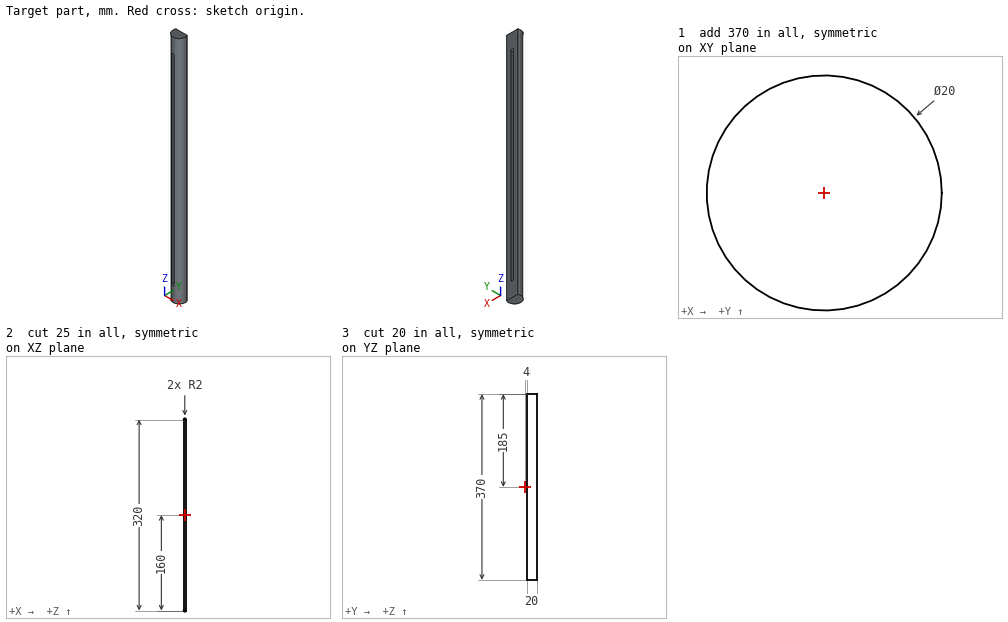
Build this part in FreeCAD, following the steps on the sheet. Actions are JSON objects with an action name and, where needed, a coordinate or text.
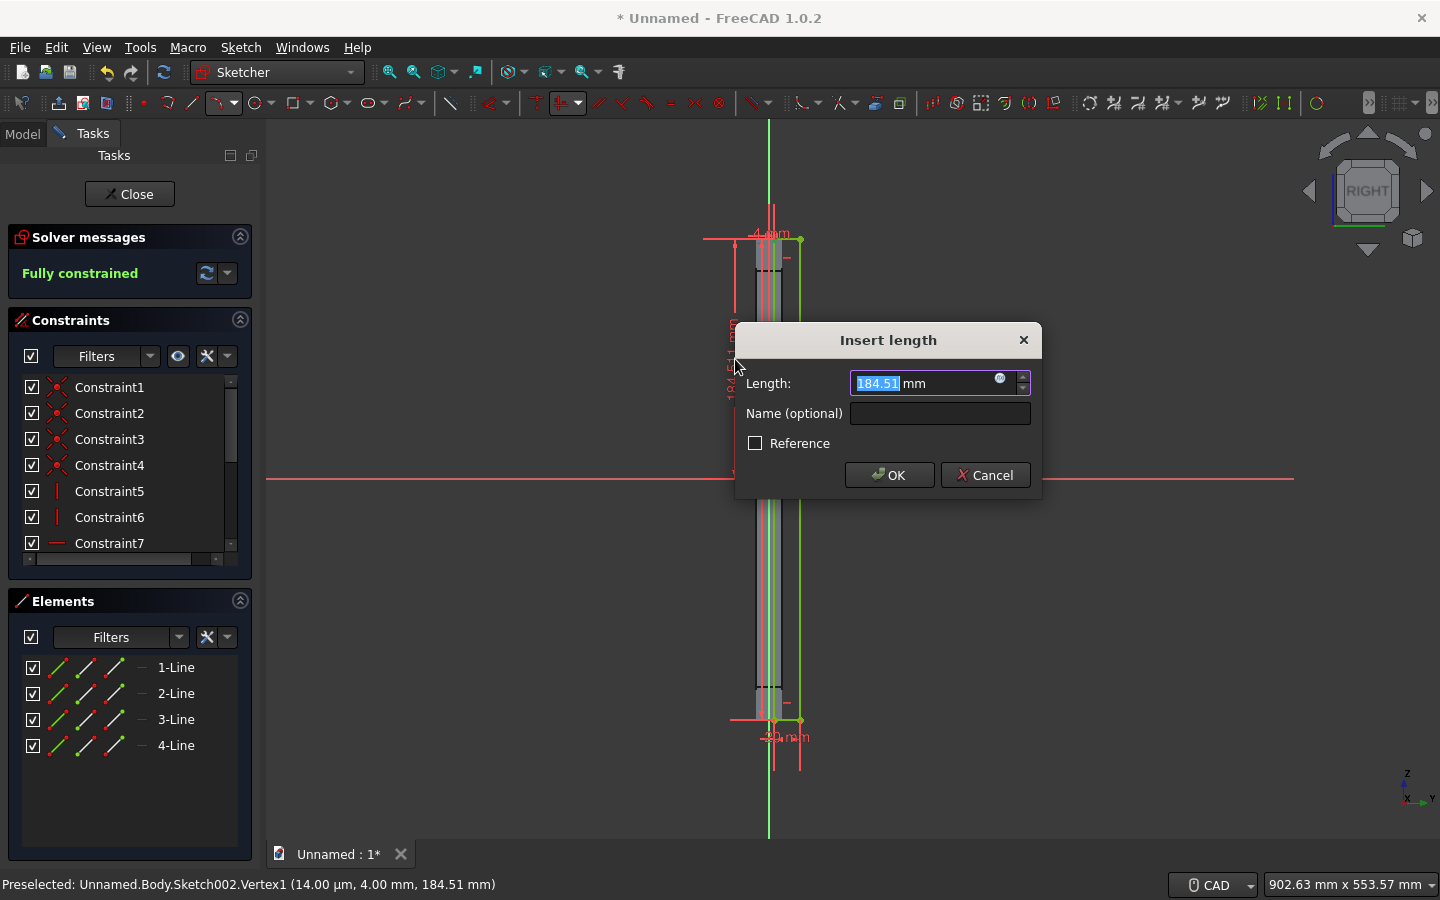
{"action": "type", "text": "185"}
{"action": "key", "text": "Return"}
{"action": "key", "text": "Escape"}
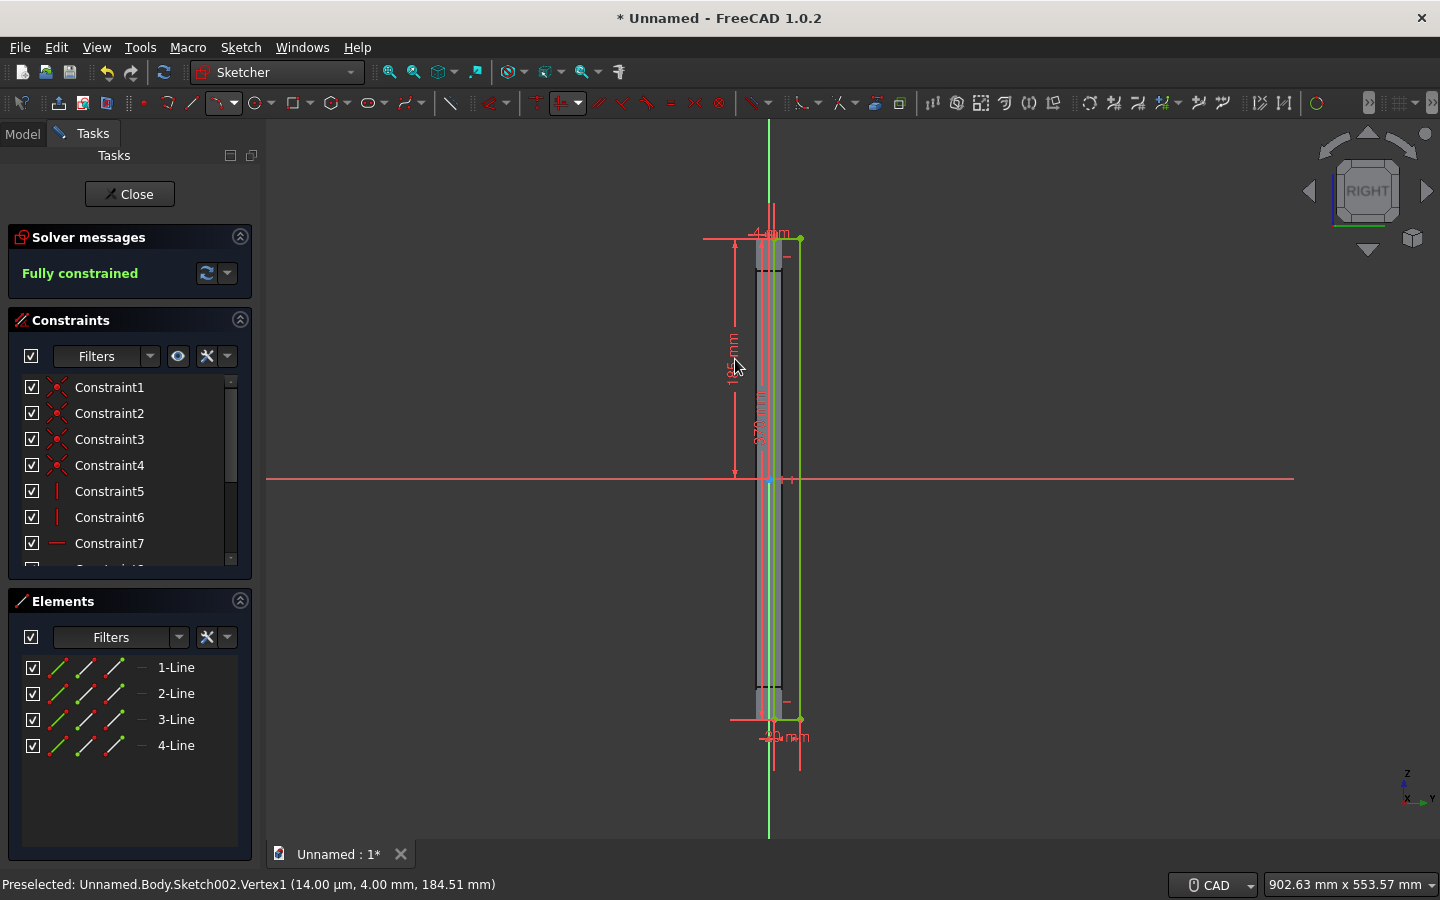
{"action": "left_click", "coordinate": [130, 194]}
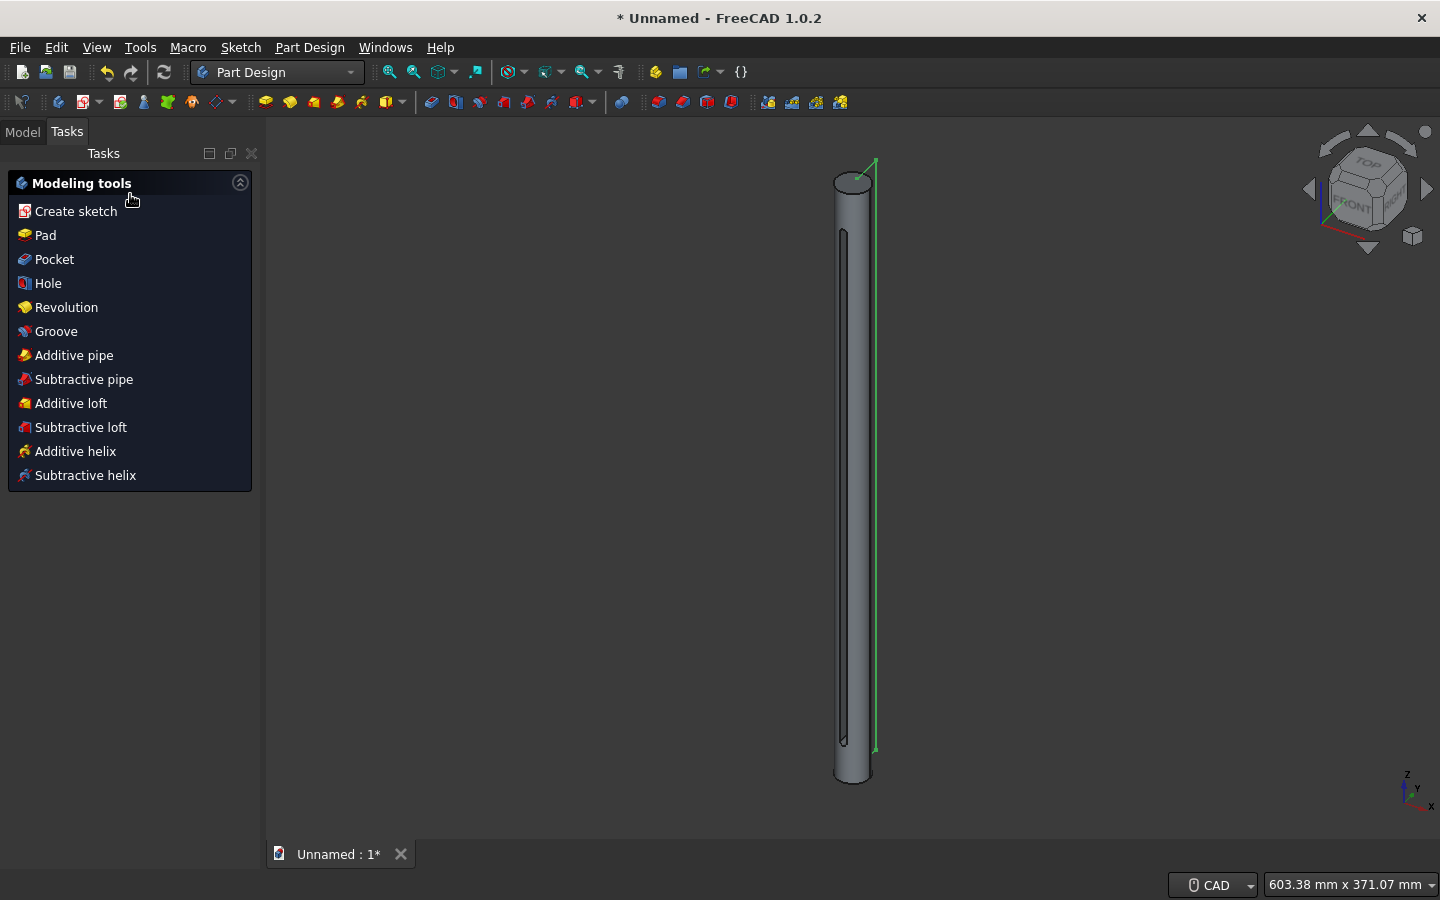
{"action": "left_click", "coordinate": [432, 102]}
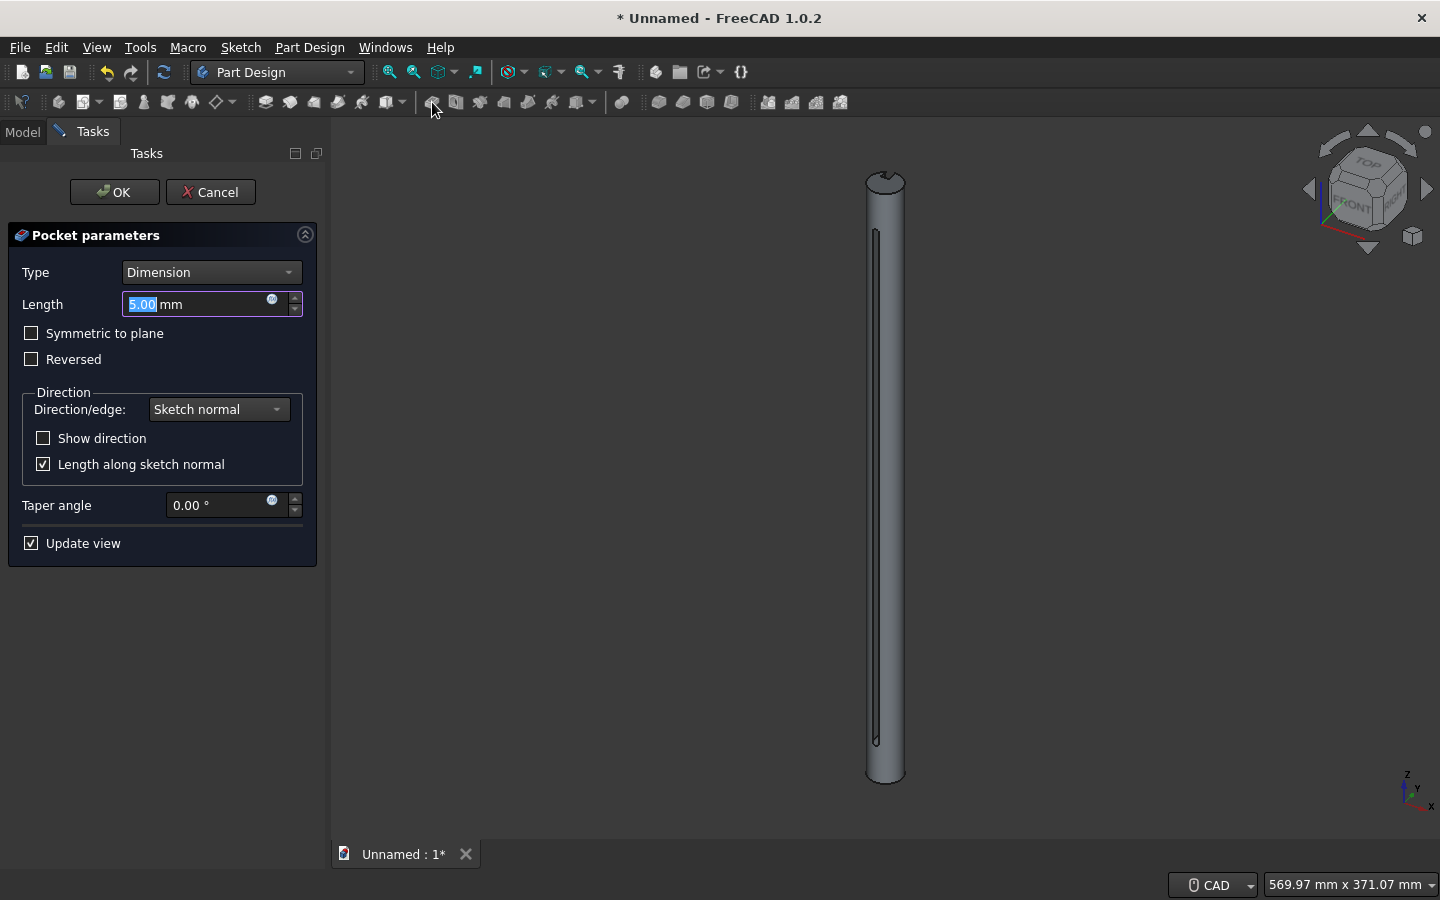
{"action": "type", "text": "20"}
{"action": "key", "text": "Tab"}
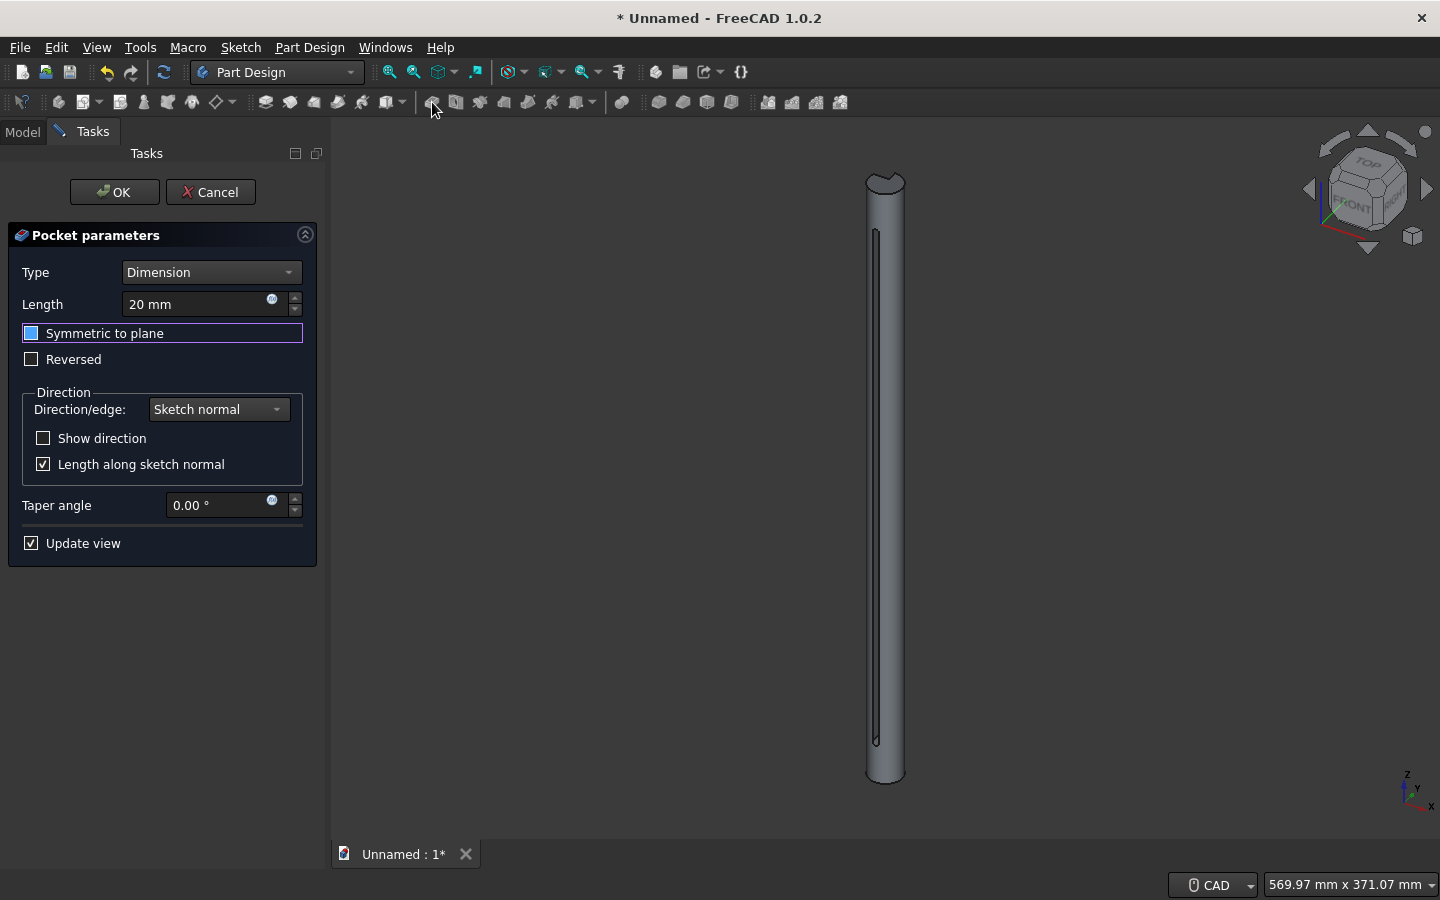
{"action": "left_click", "coordinate": [30, 333]}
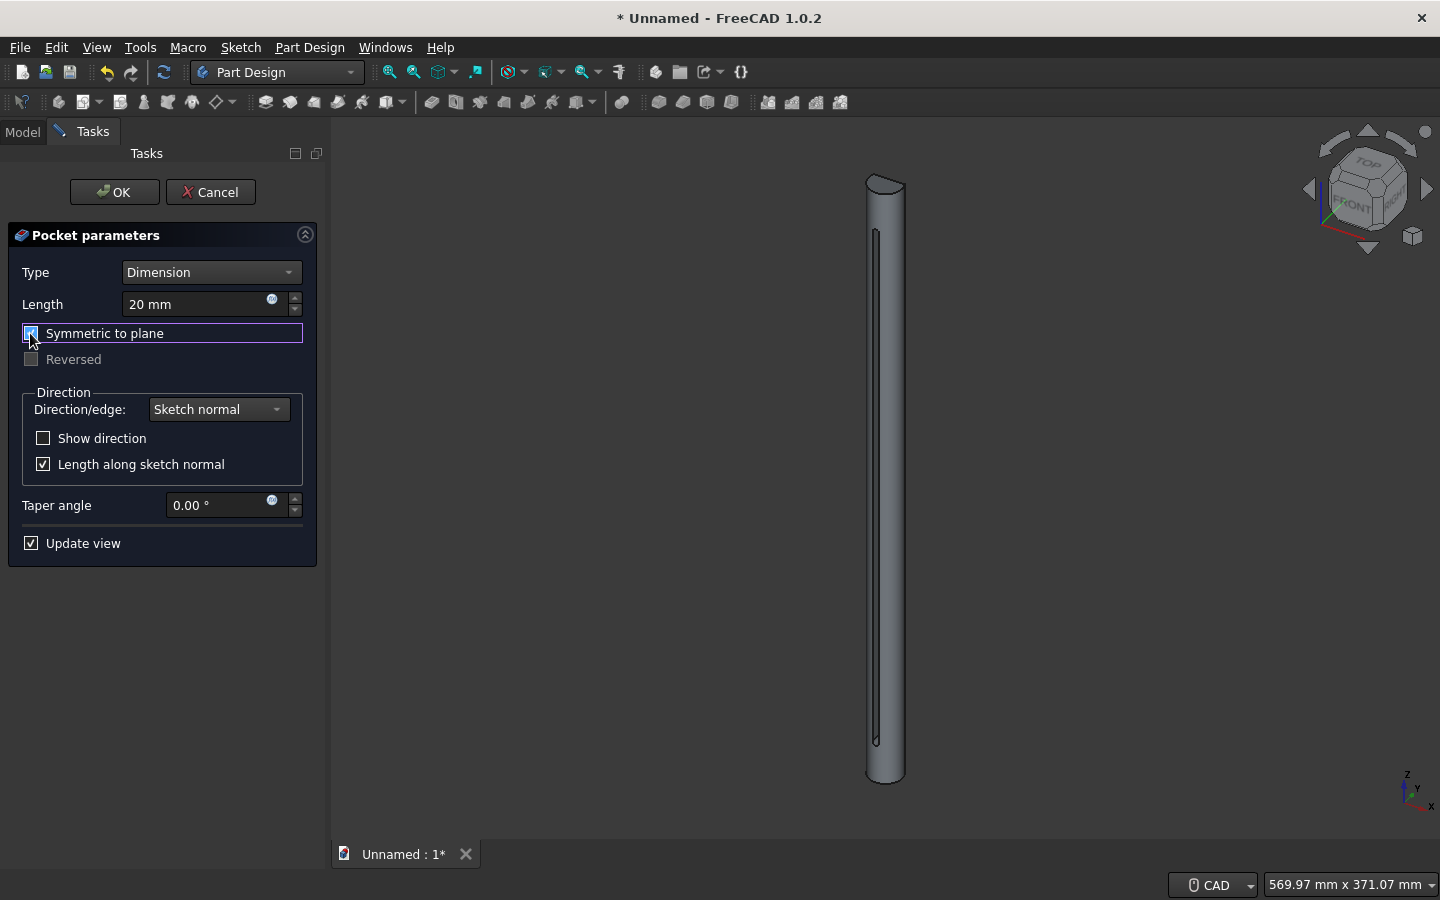
{"action": "left_click", "coordinate": [115, 192]}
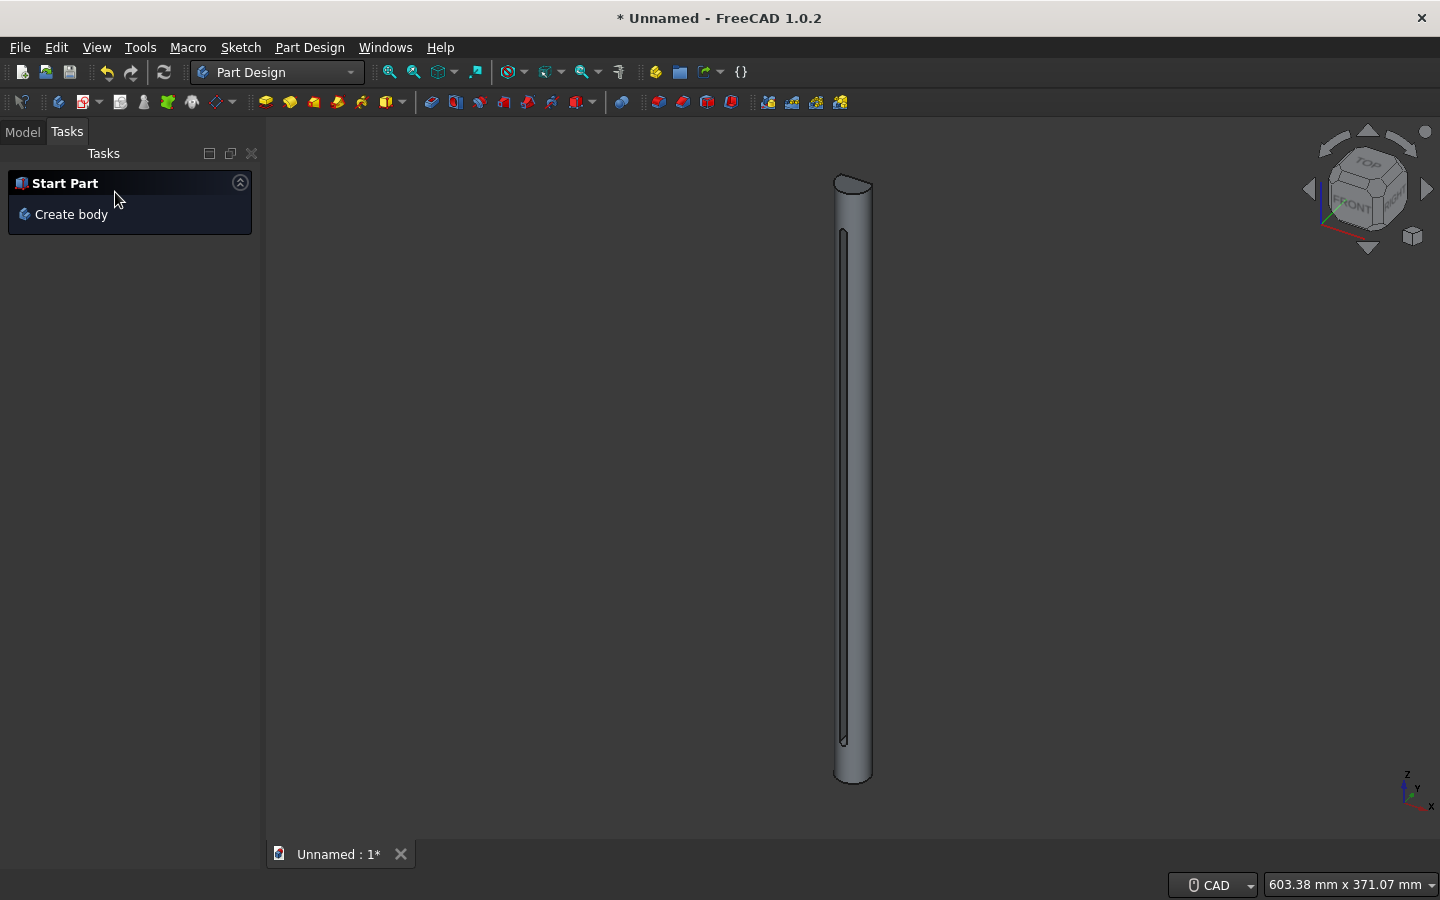
{"action": "key", "text": "0"}